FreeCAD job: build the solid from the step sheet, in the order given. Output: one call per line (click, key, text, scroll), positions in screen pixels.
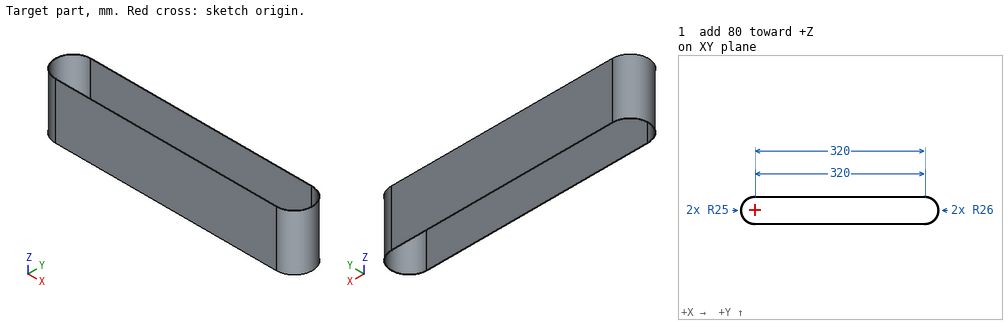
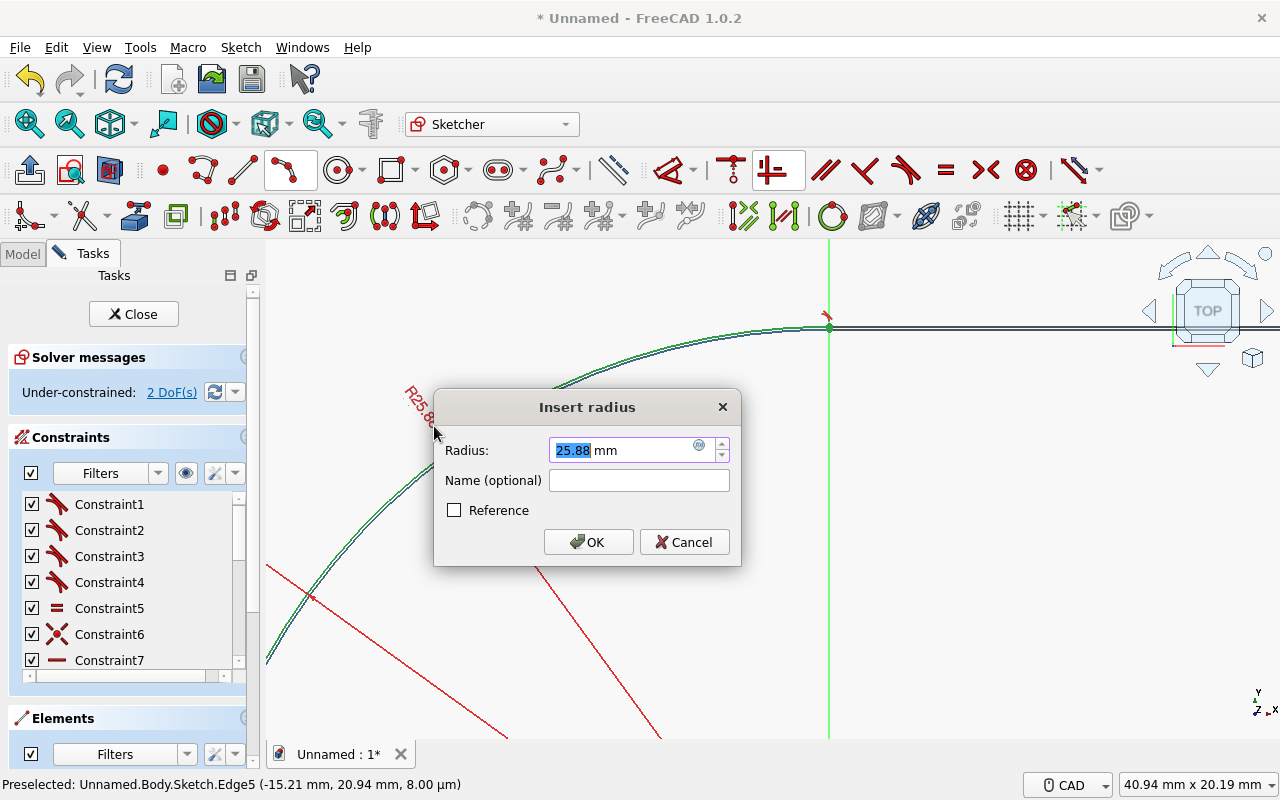
text(25)
key(Return)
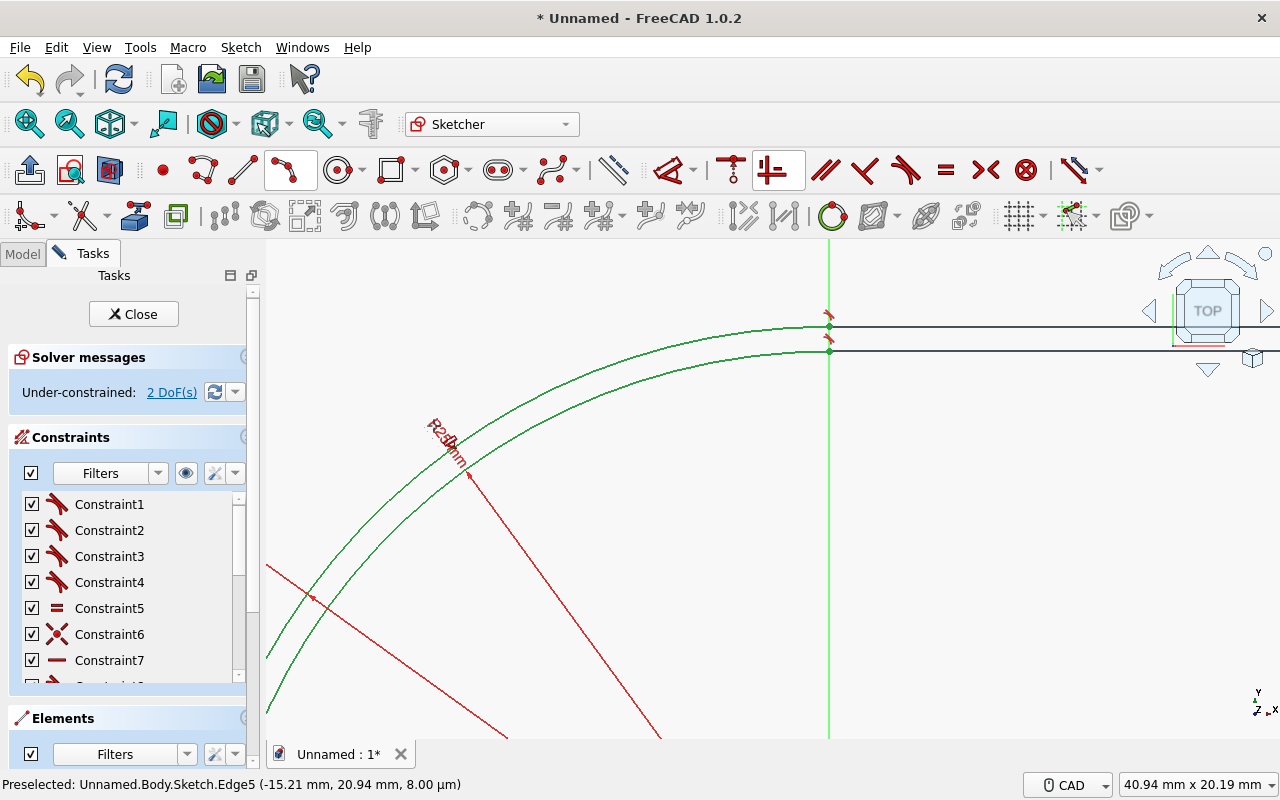
scroll(440, 458, down, 14)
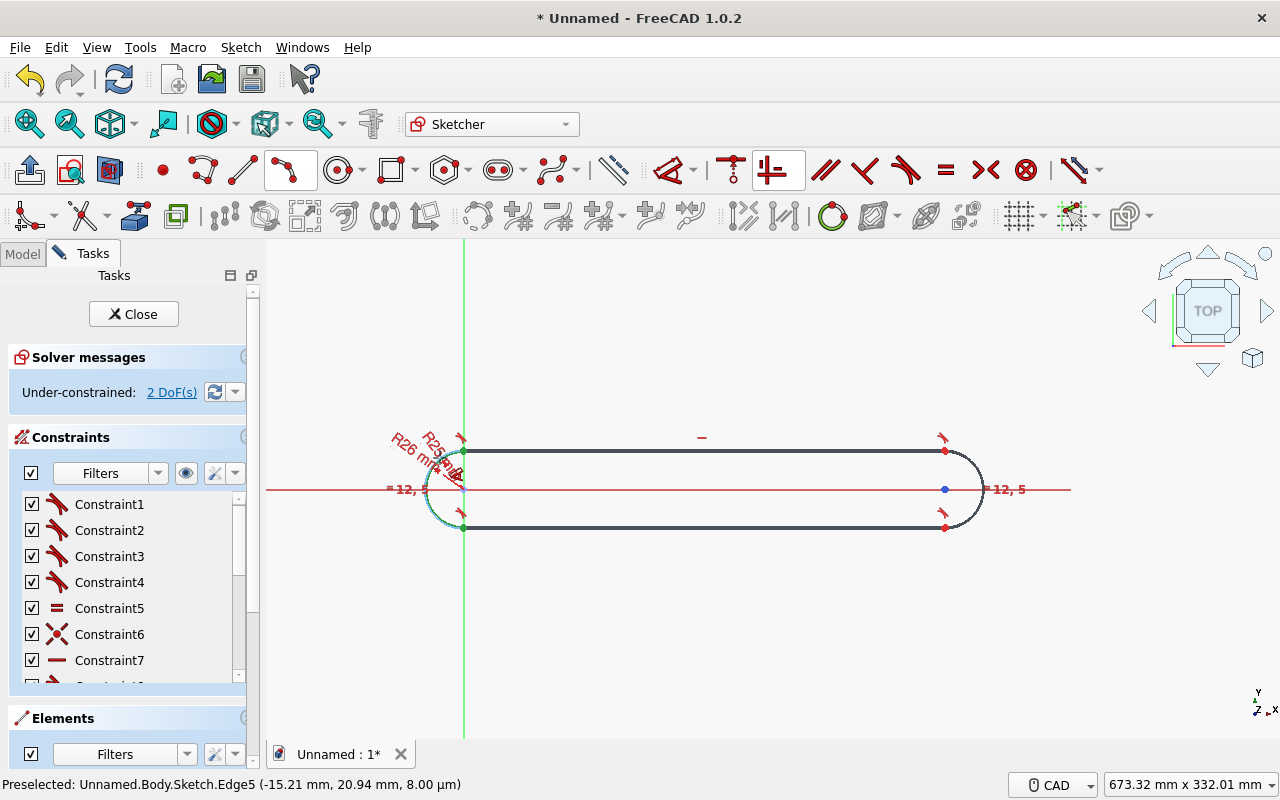
scroll(608, 450, up, 12)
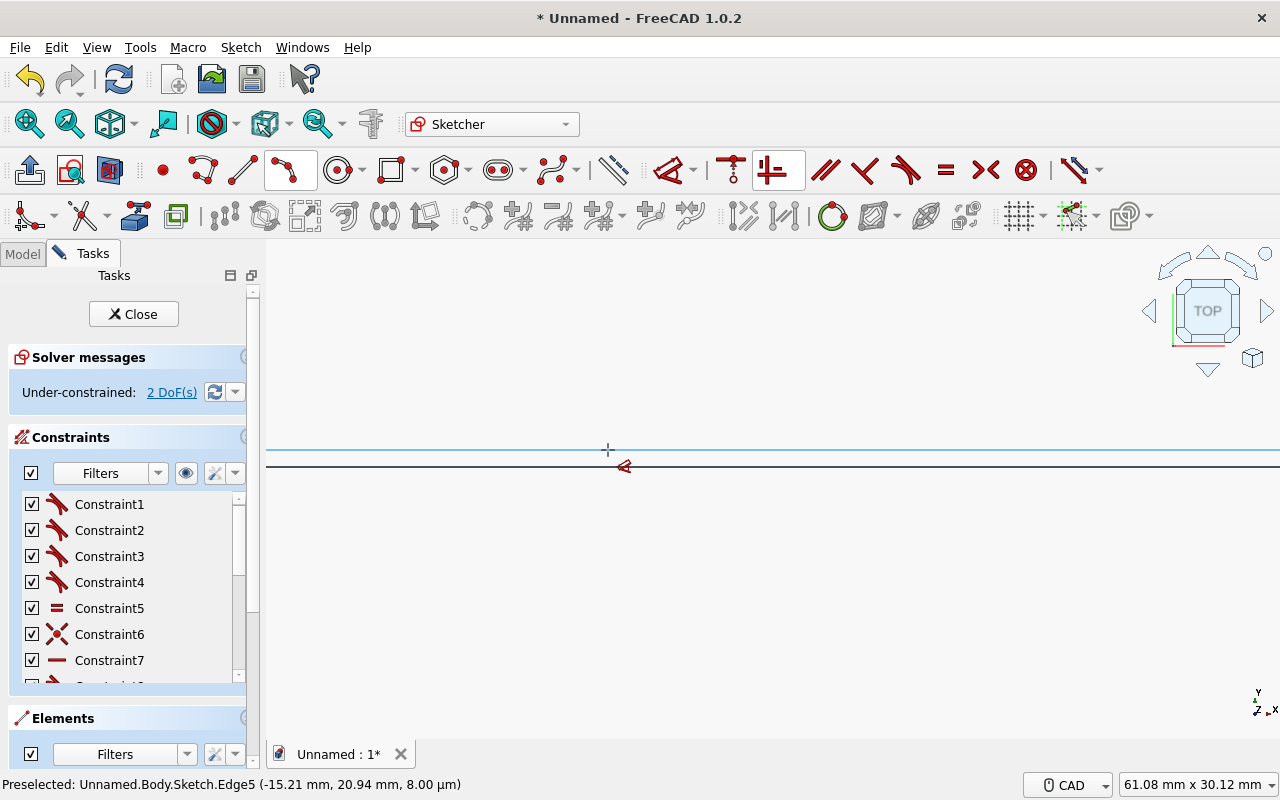
click(605, 450)
click(704, 416)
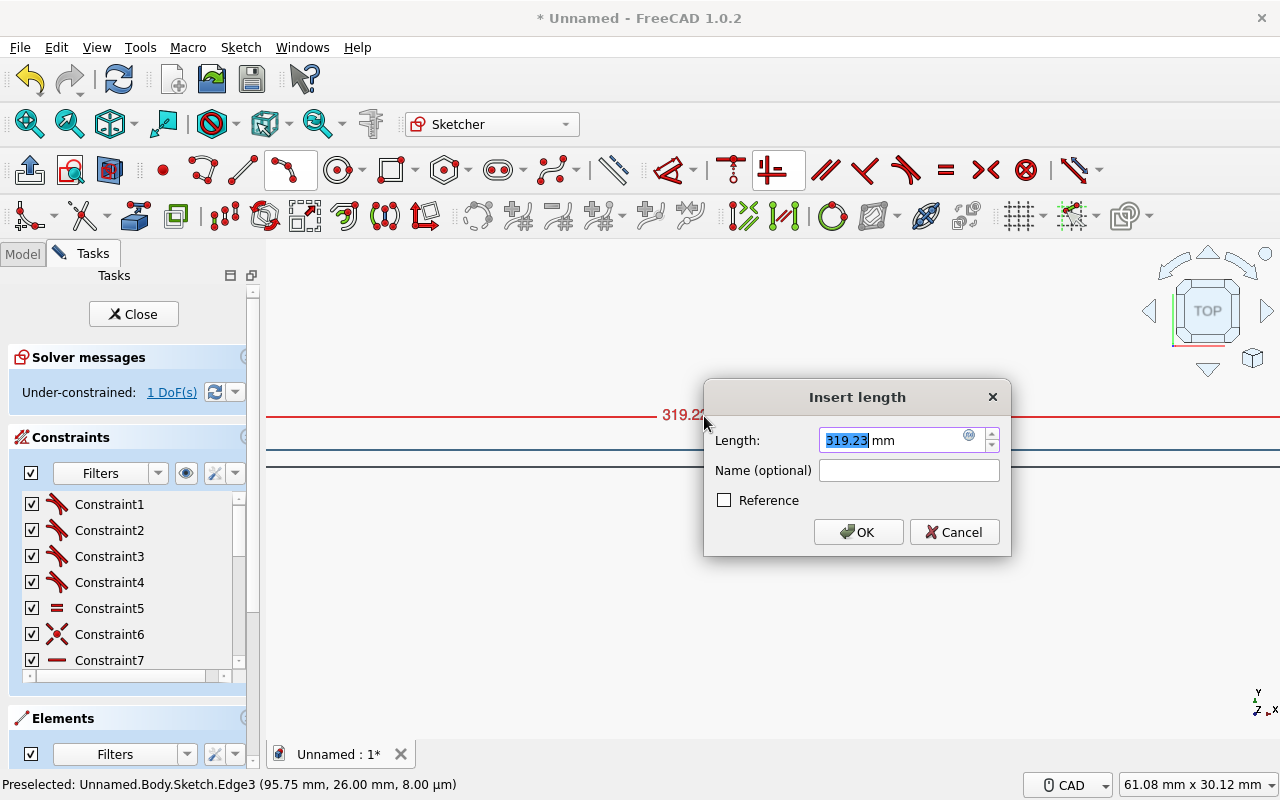
text(320)
key(Return)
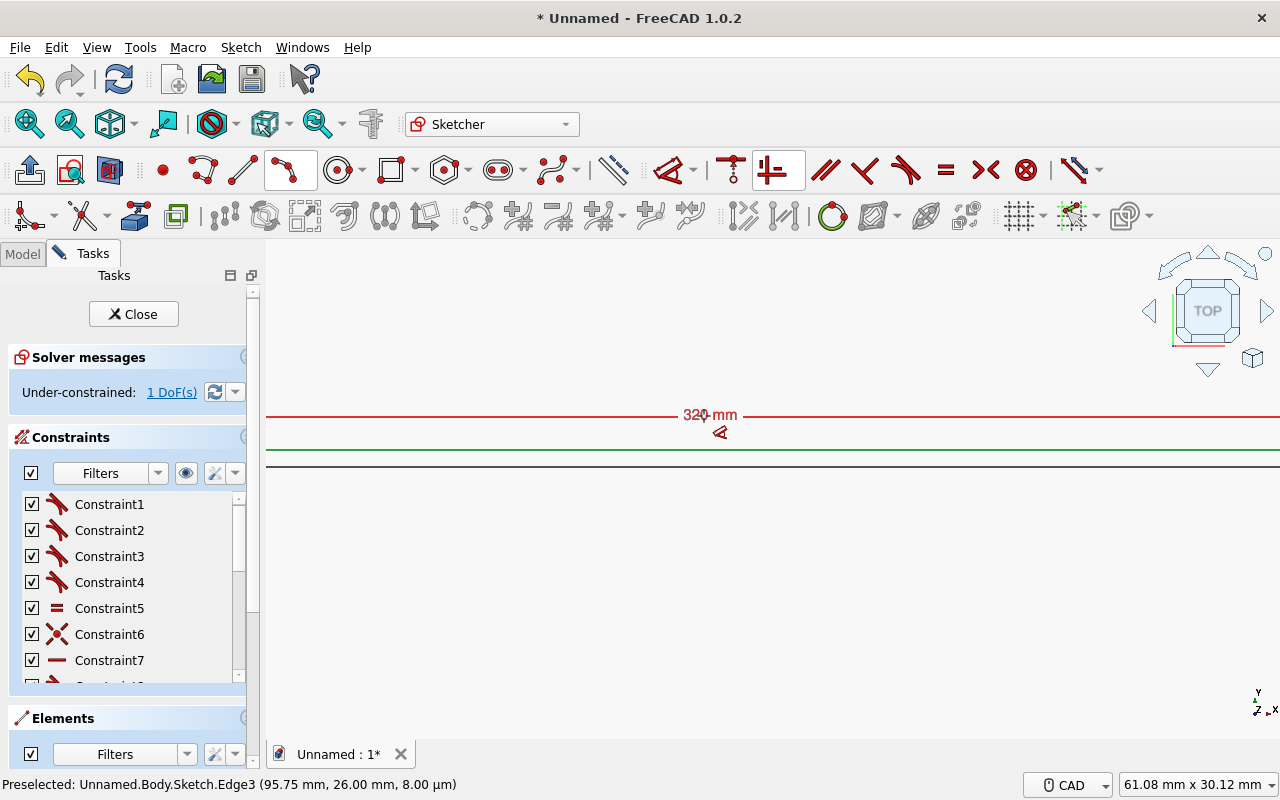
click(608, 467)
click(516, 433)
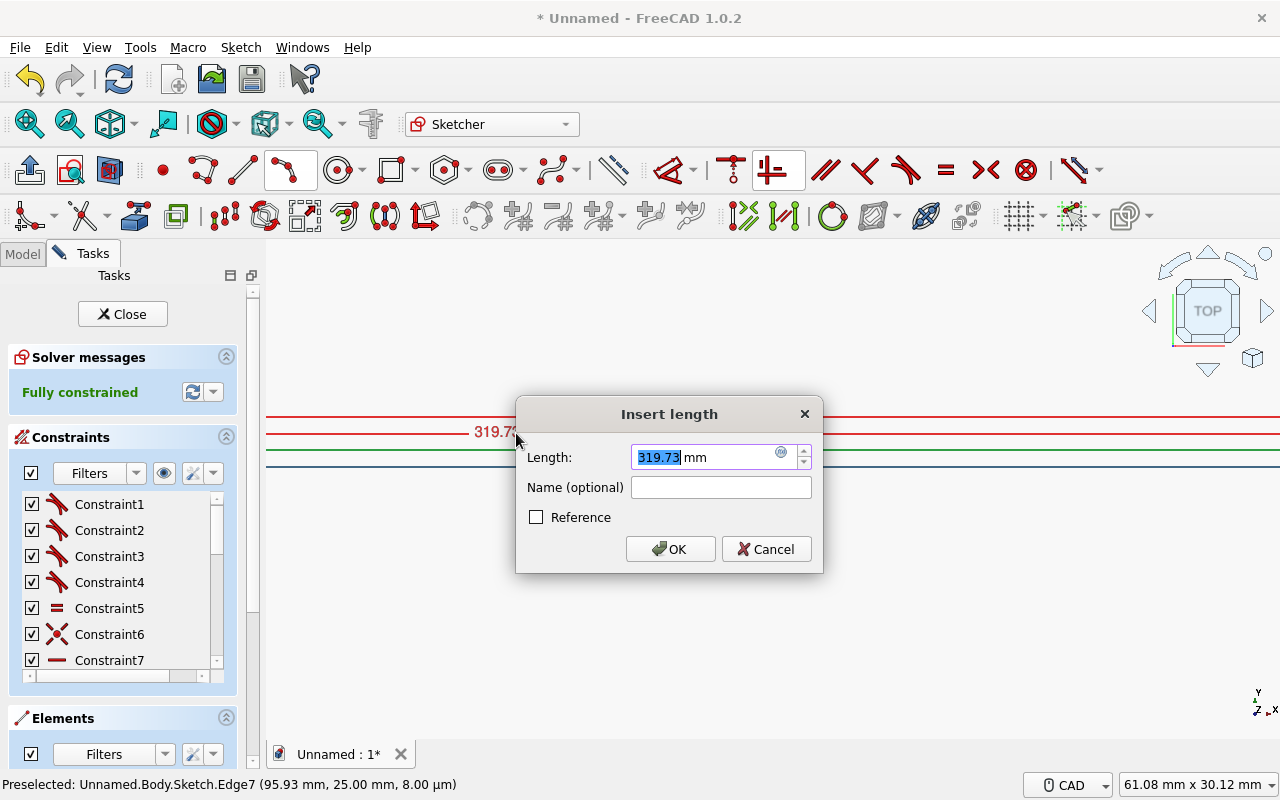
text(320)
key(Return)
key(Escape)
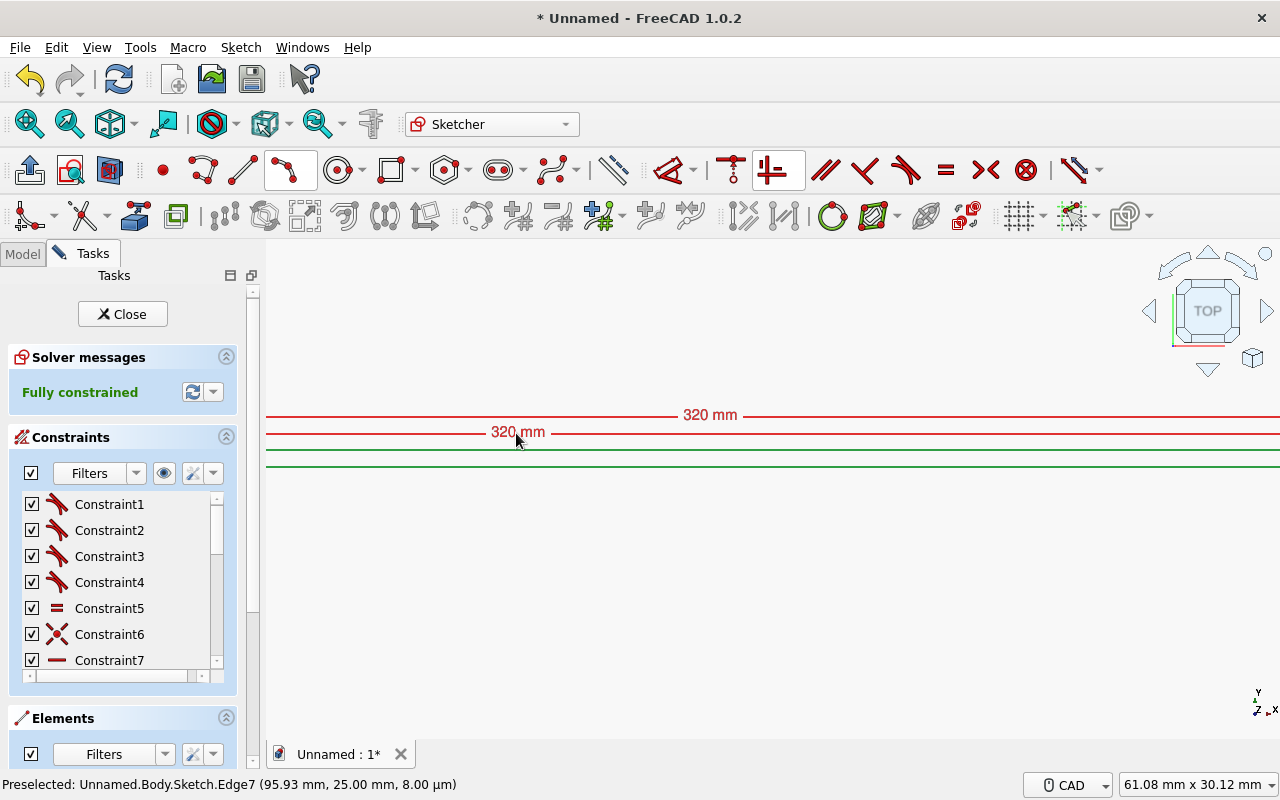
click(123, 314)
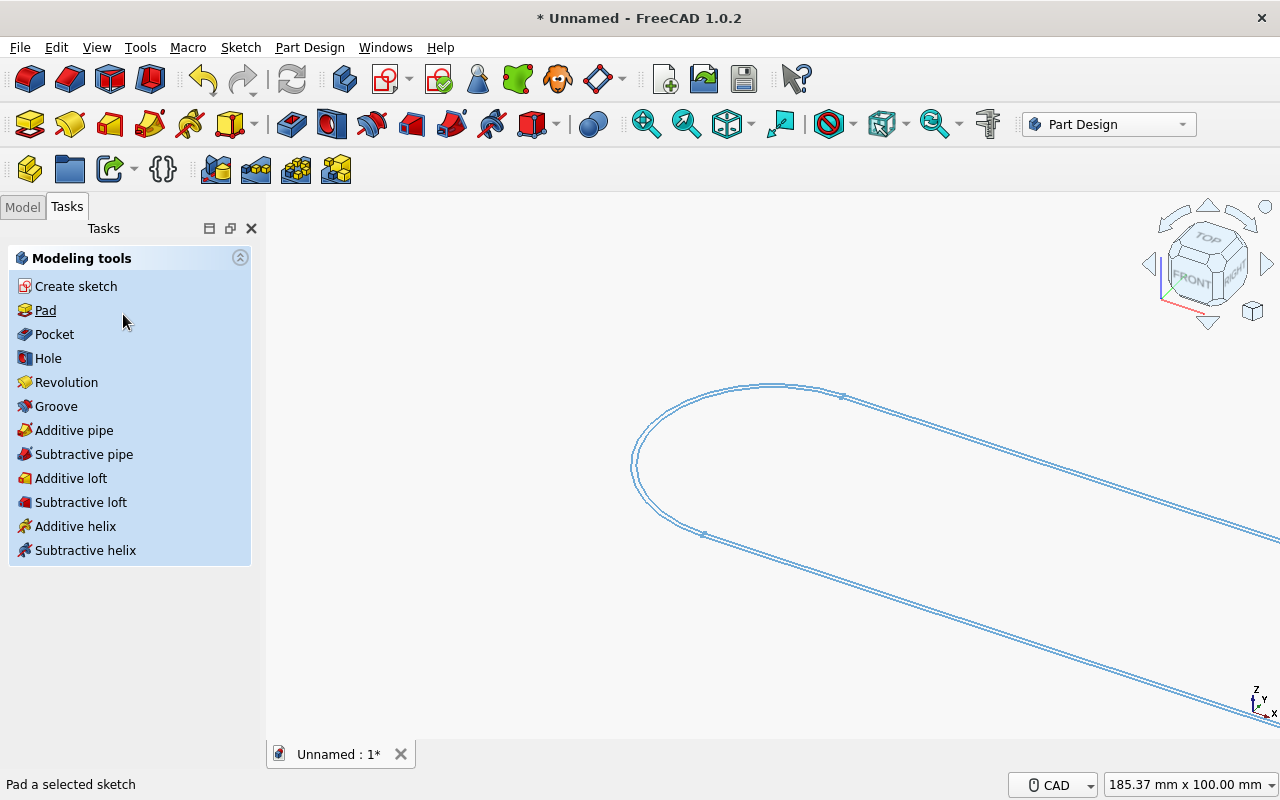
click(30, 124)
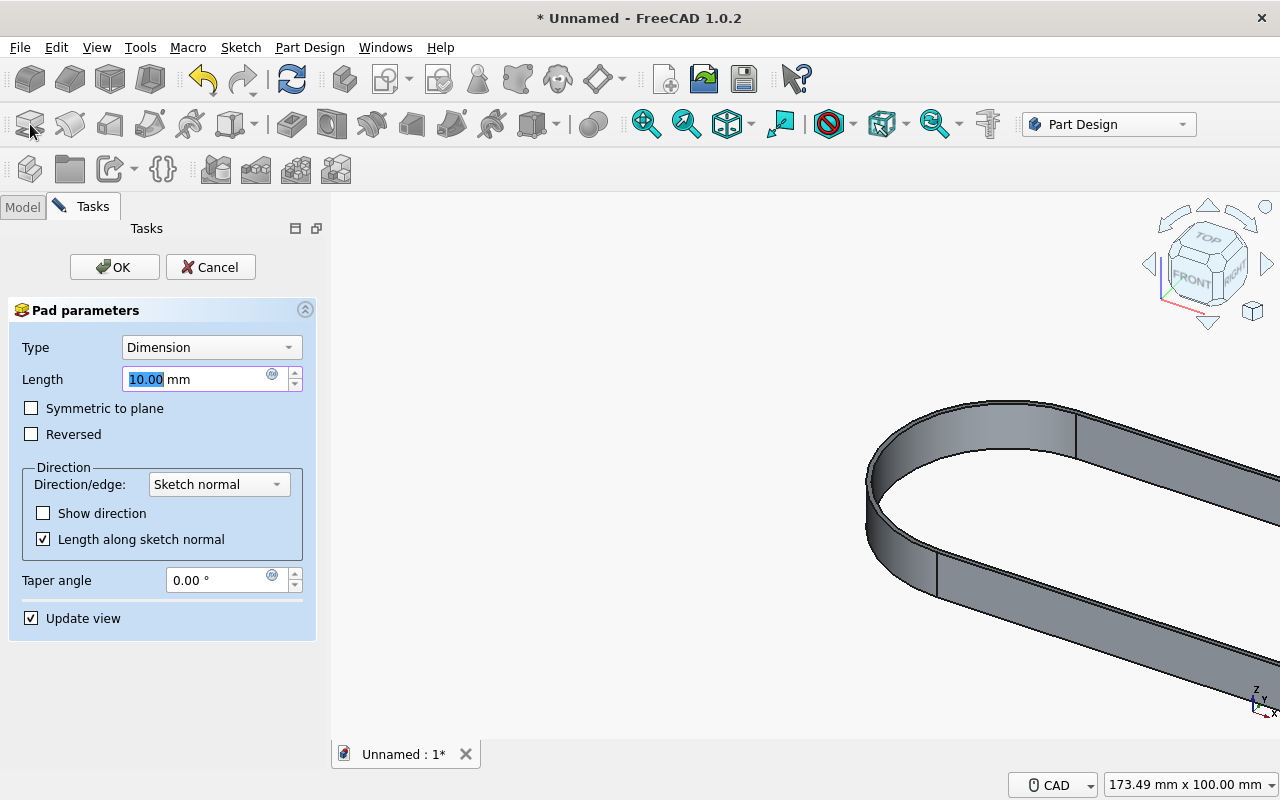
text(80)
key(Tab)